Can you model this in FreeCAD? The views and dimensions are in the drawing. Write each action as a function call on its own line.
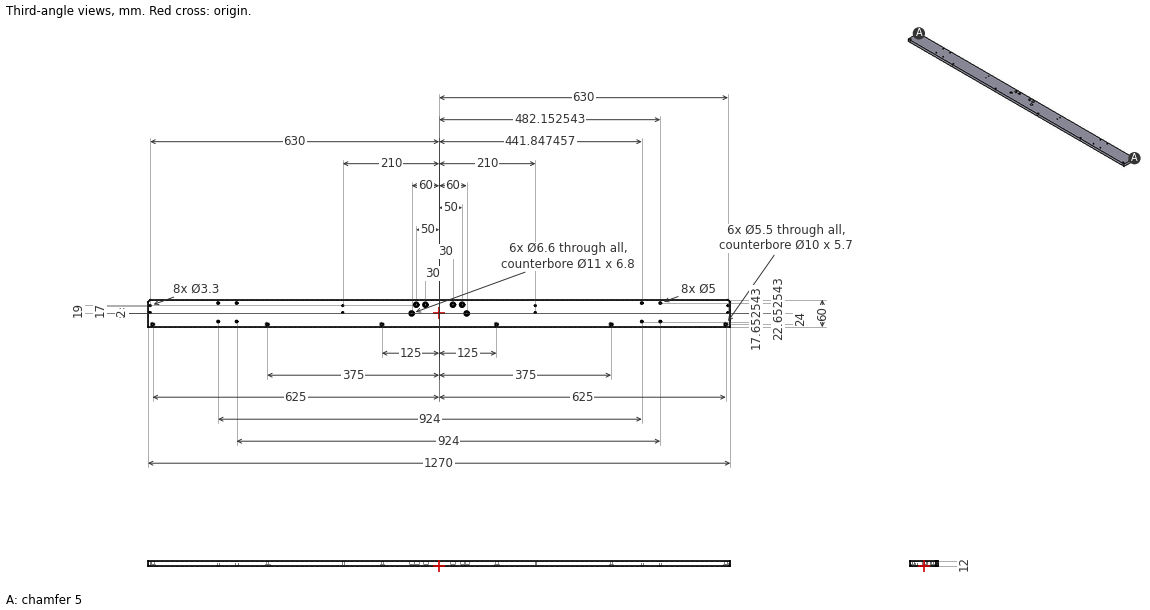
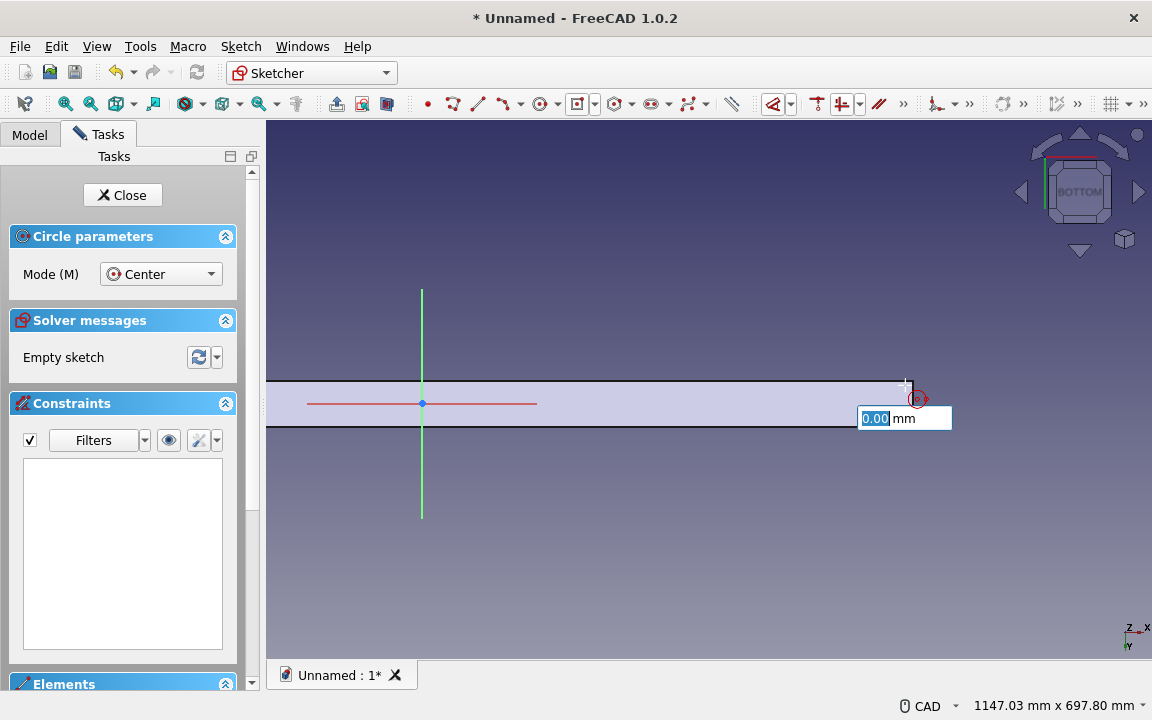
scroll(907, 384, up, 11)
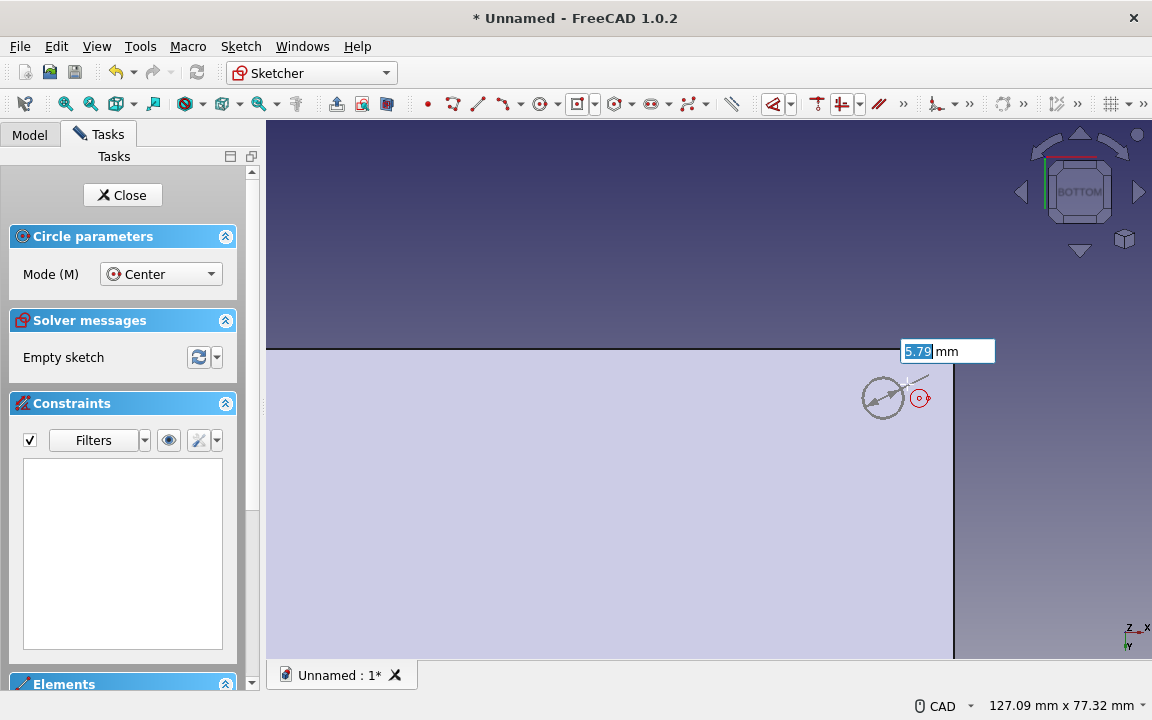
click(898, 377)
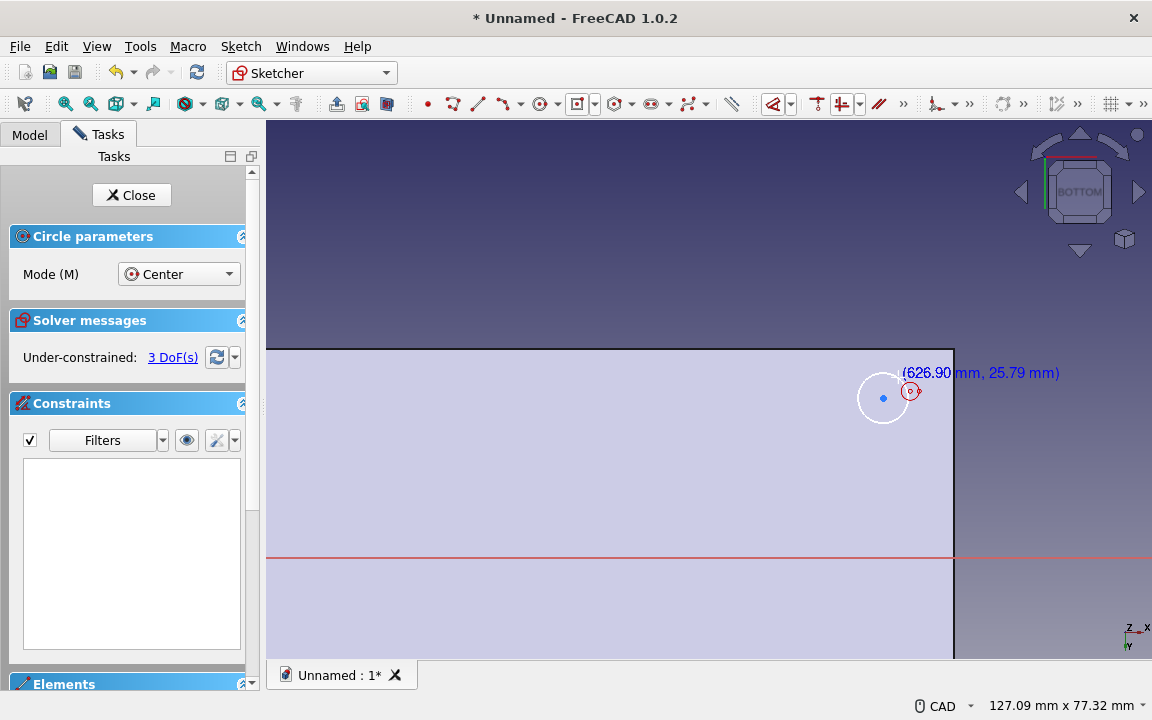
scroll(907, 385, down, 14)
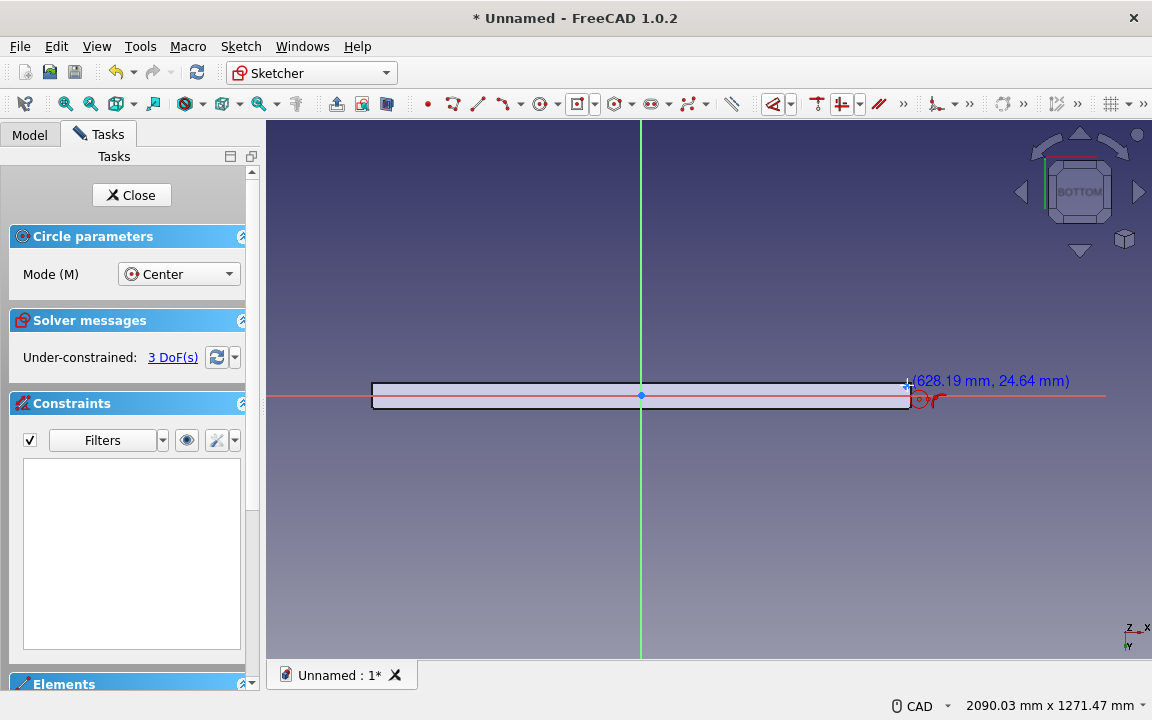
scroll(800, 386, up, 15)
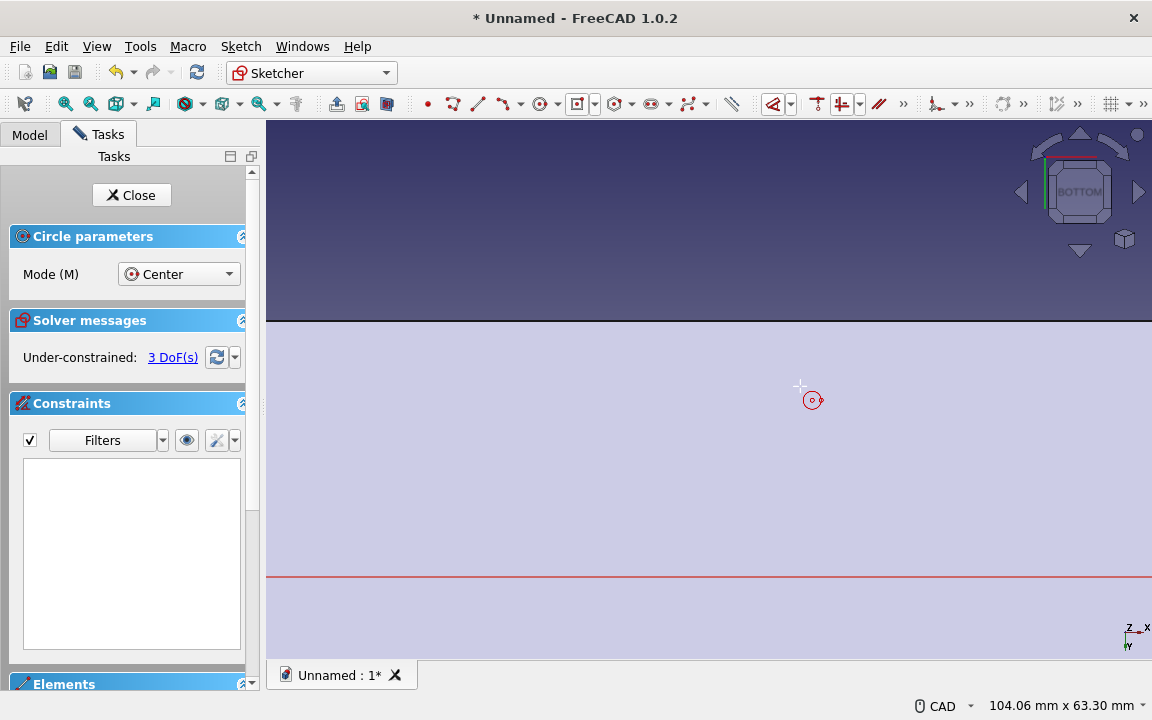
scroll(800, 386, down, 15)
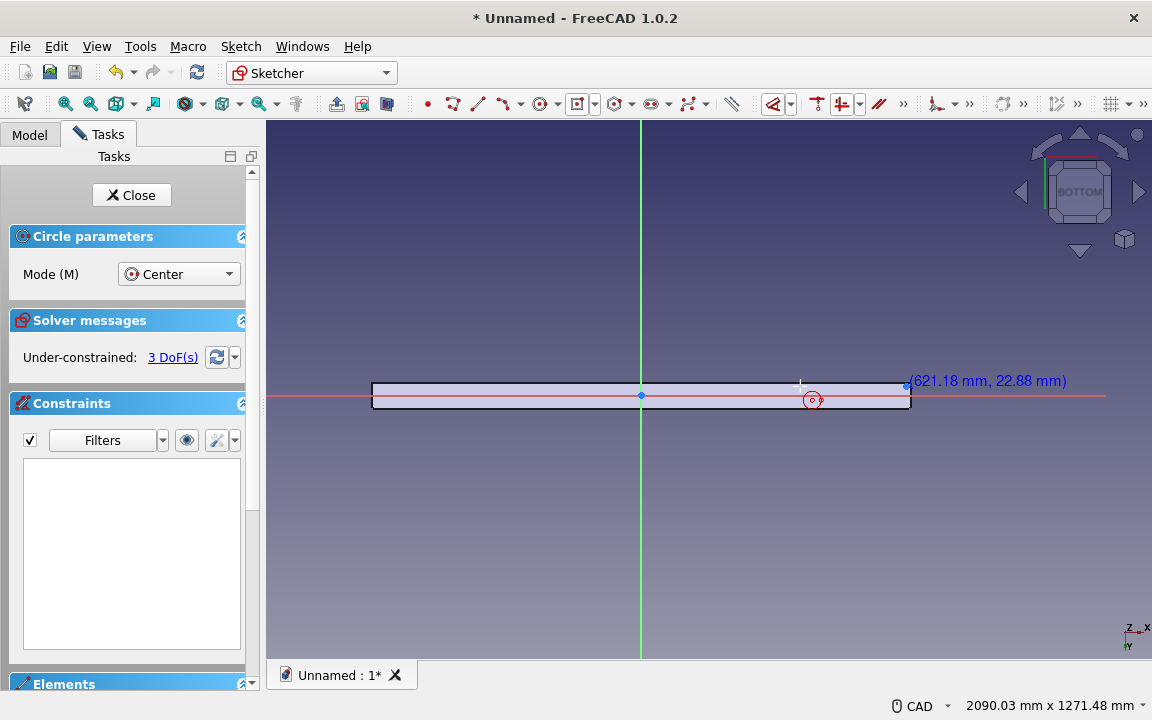
scroll(800, 386, up, 3)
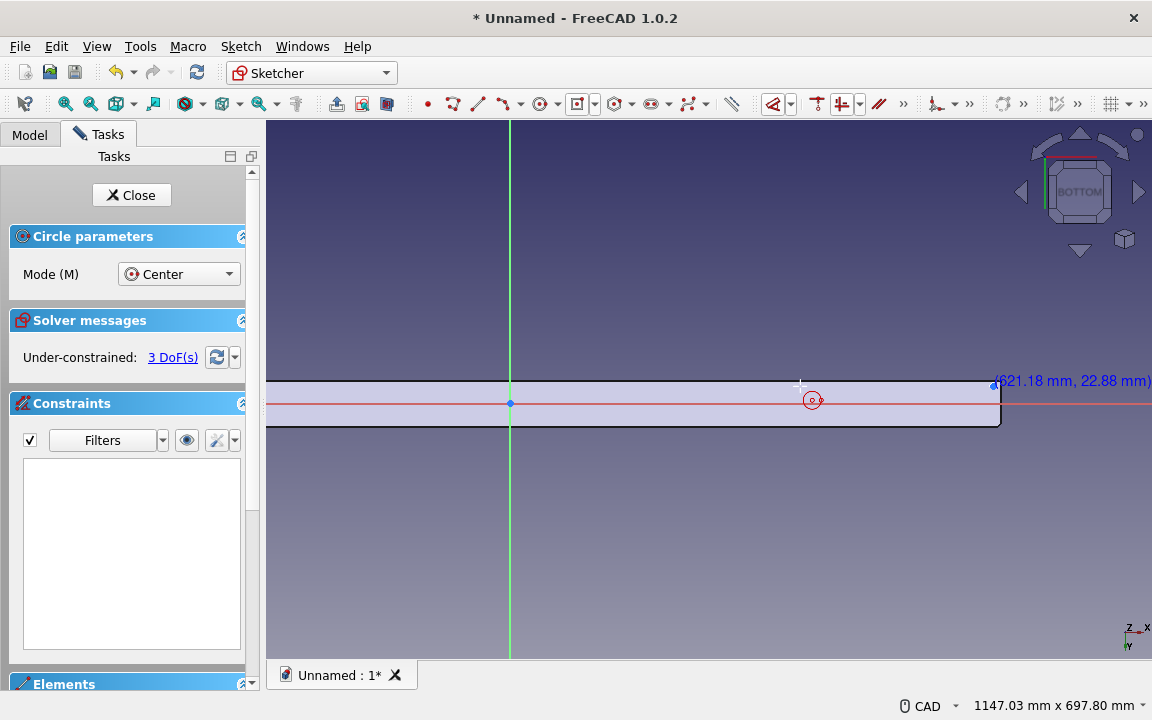
click(800, 385)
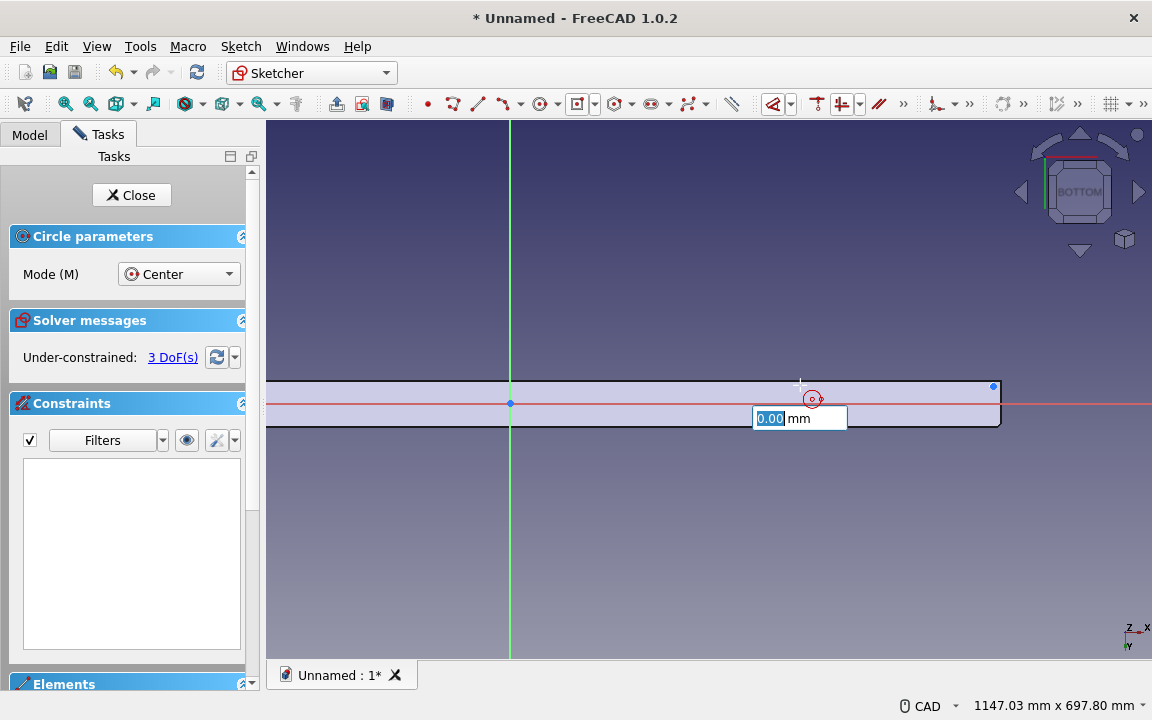
scroll(802, 384, up, 11)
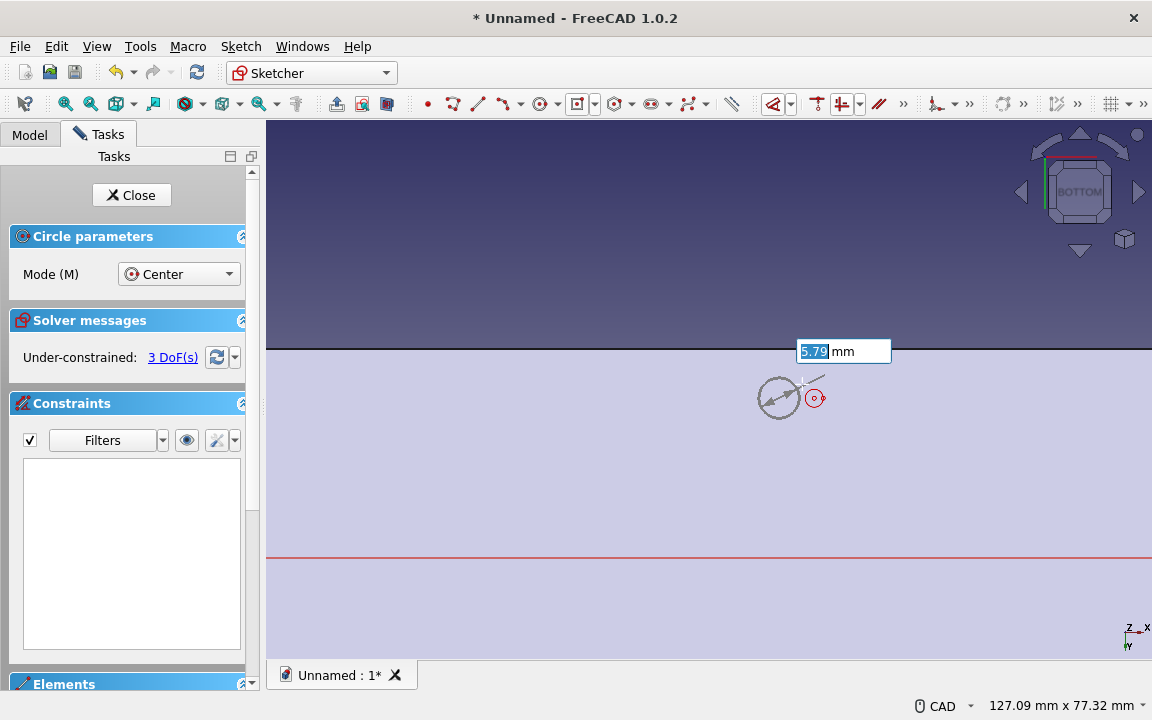
click(794, 378)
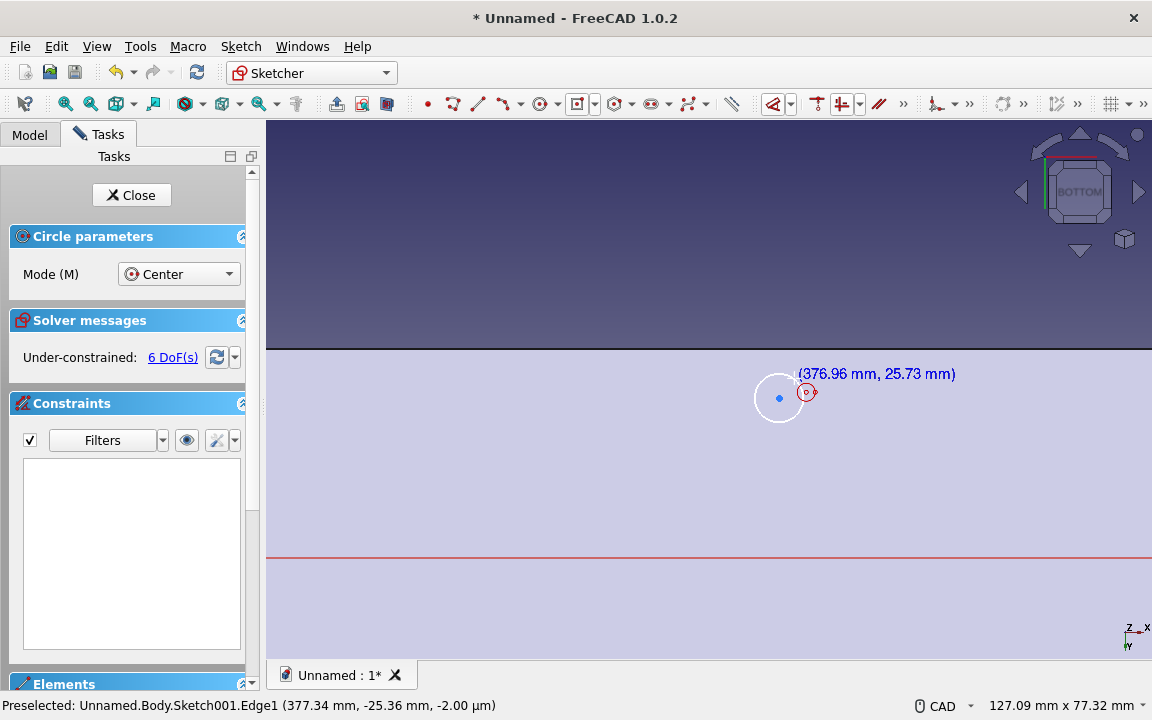
scroll(801, 385, down, 14)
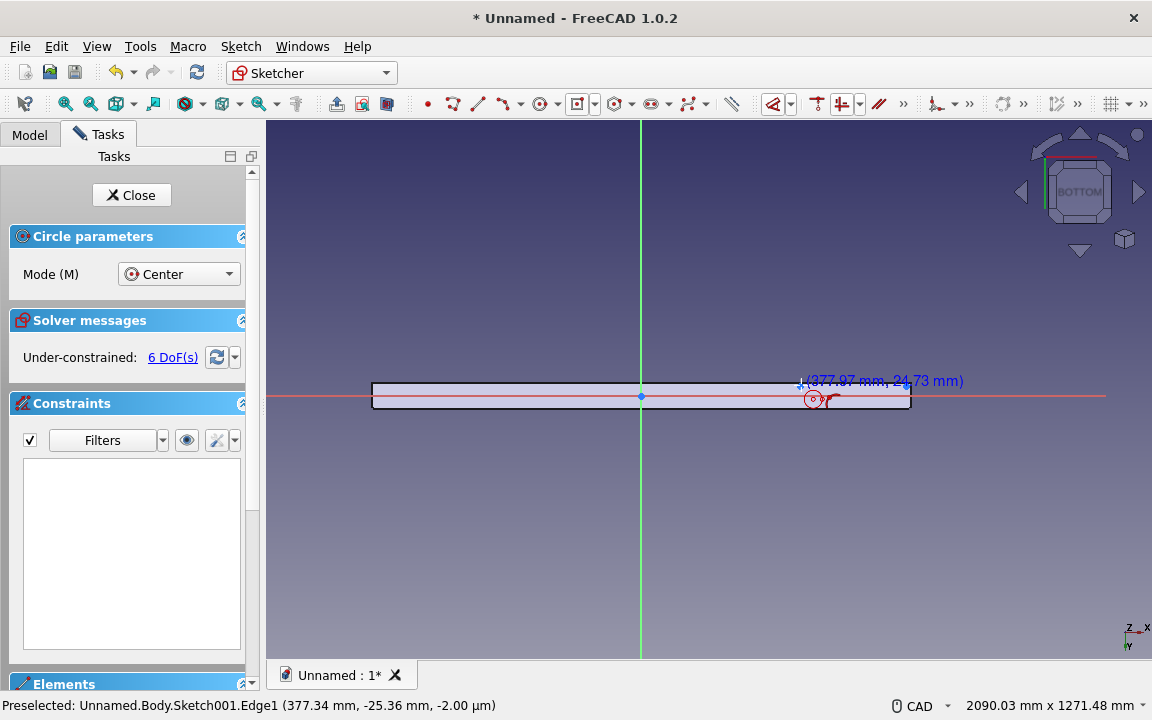
scroll(694, 386, up, 15)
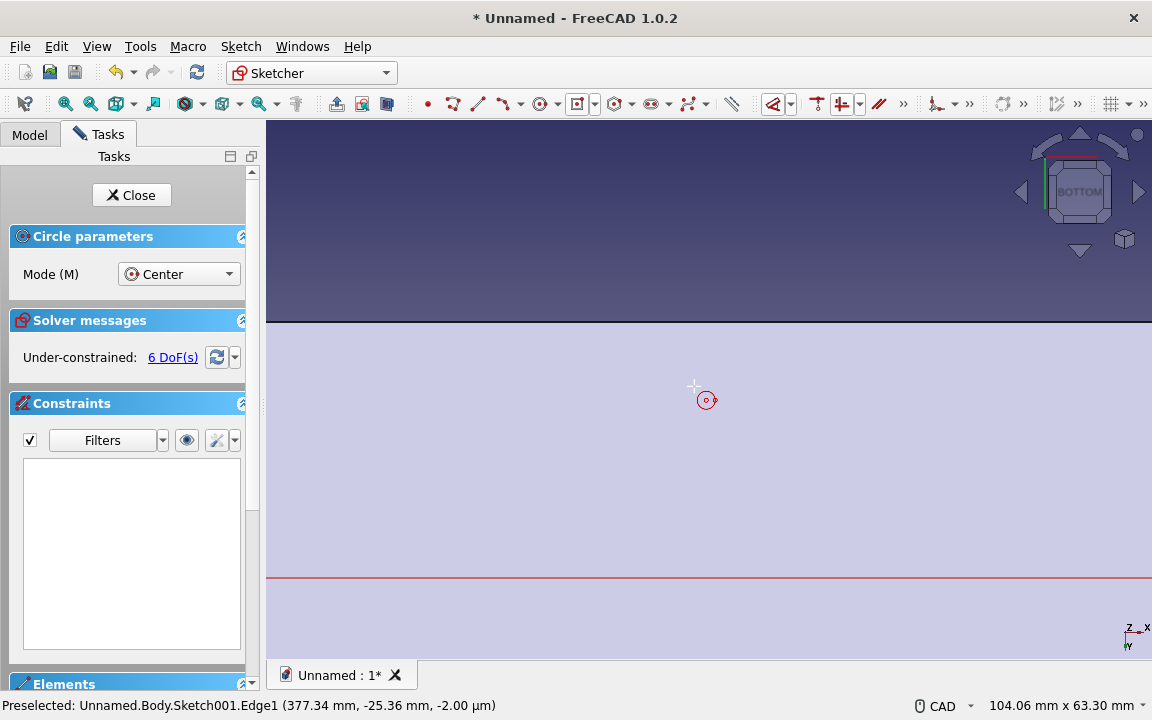
scroll(694, 386, down, 15)